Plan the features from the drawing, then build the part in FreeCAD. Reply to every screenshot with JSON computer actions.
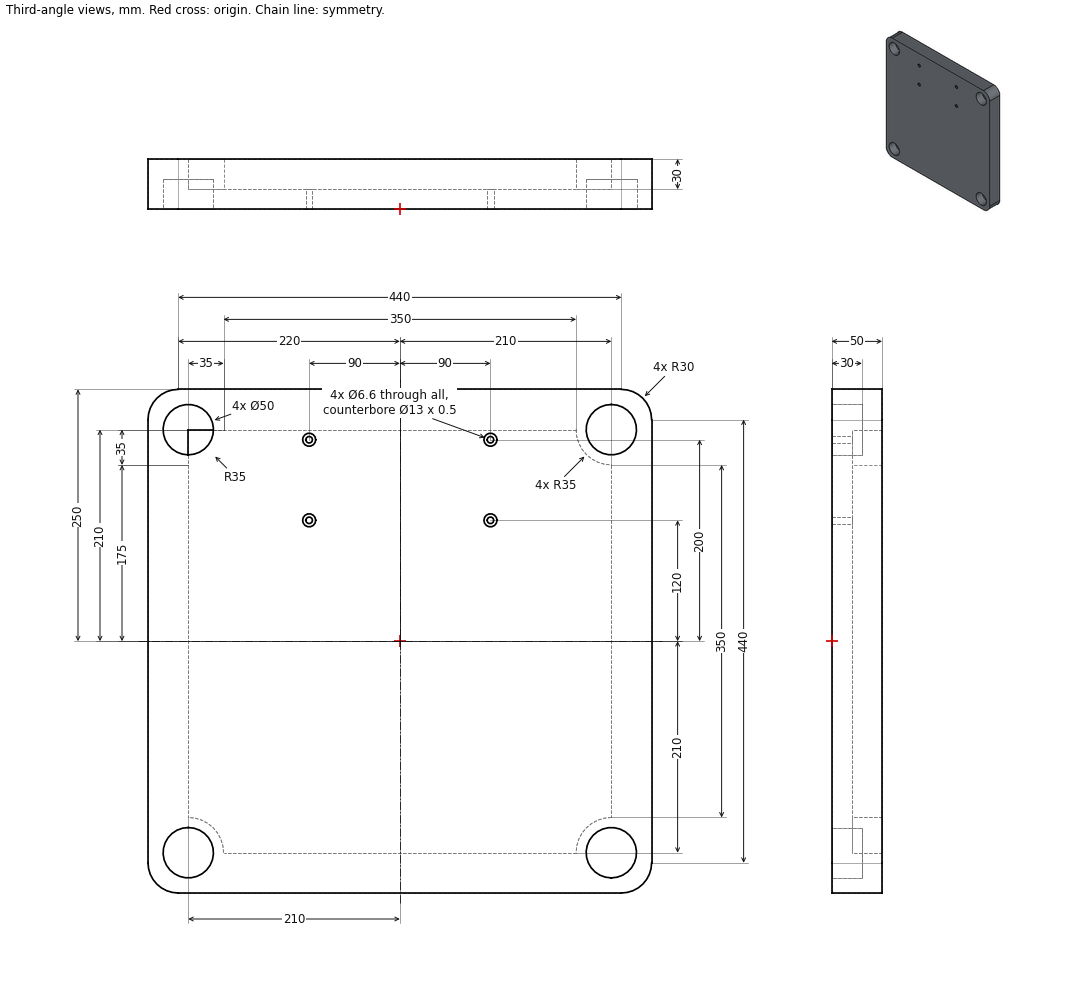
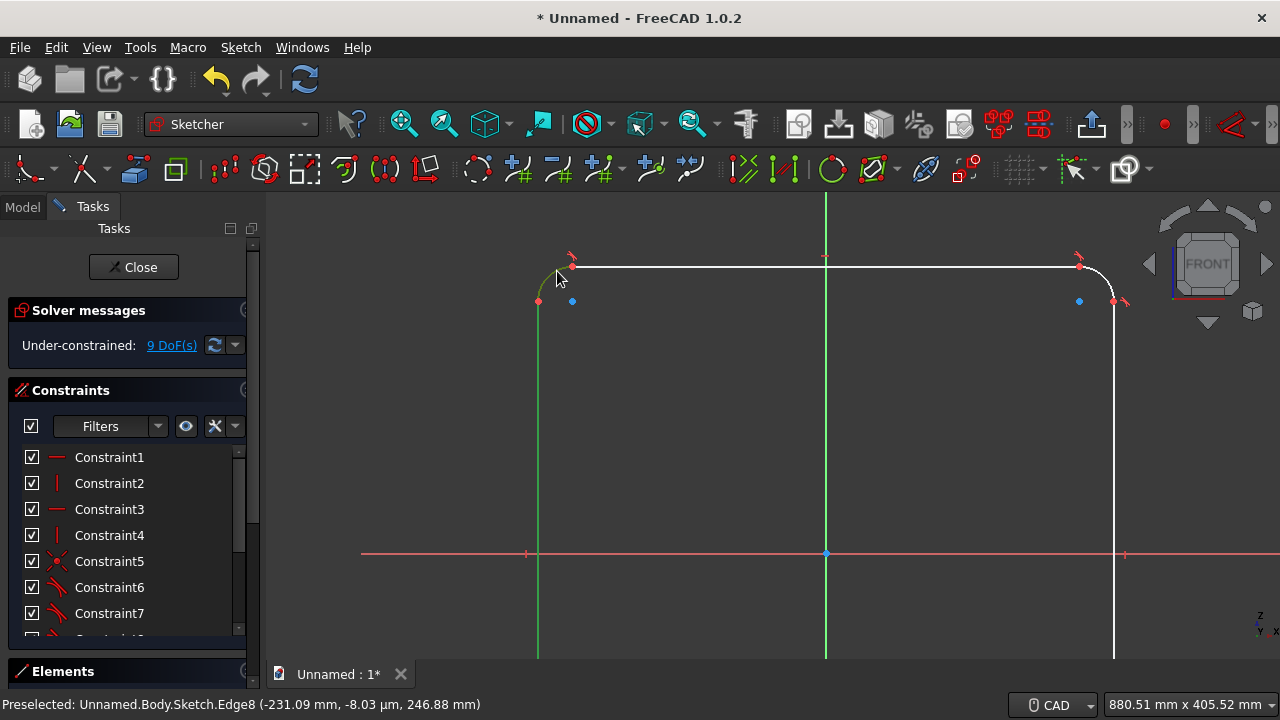
{"action": "key", "text": "t"}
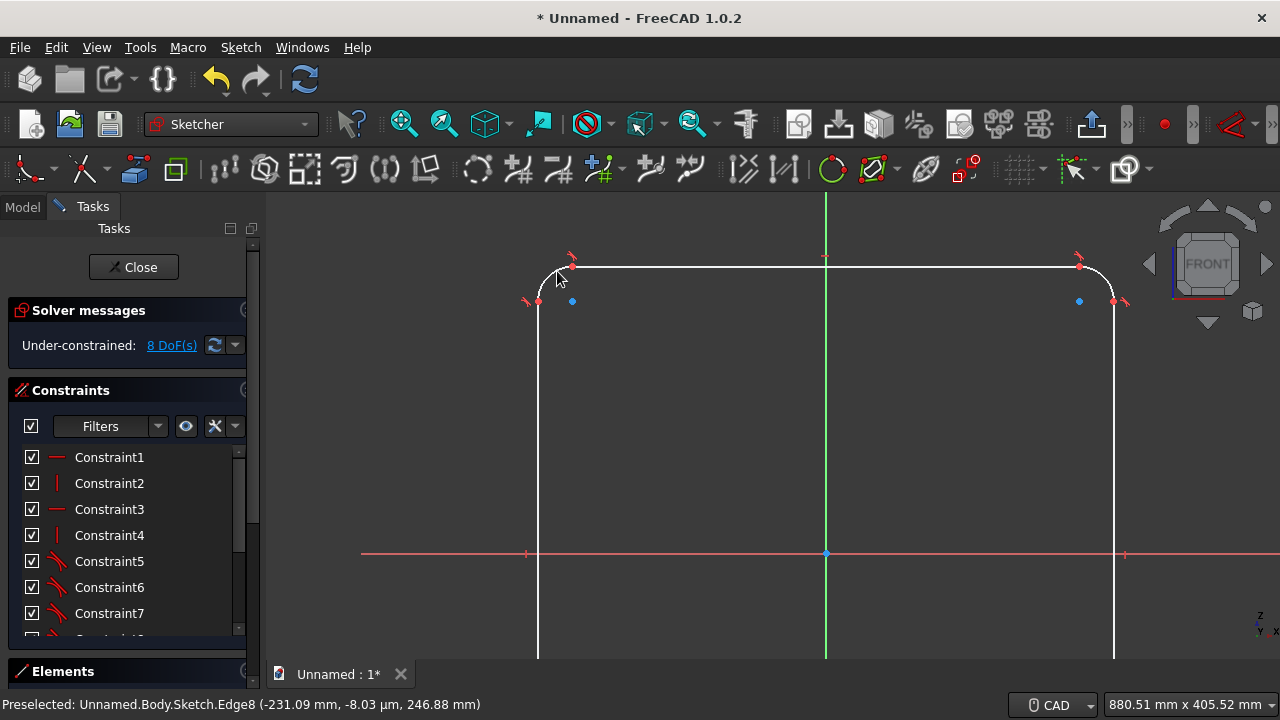
{"action": "left_click", "coordinate": [1110, 286]}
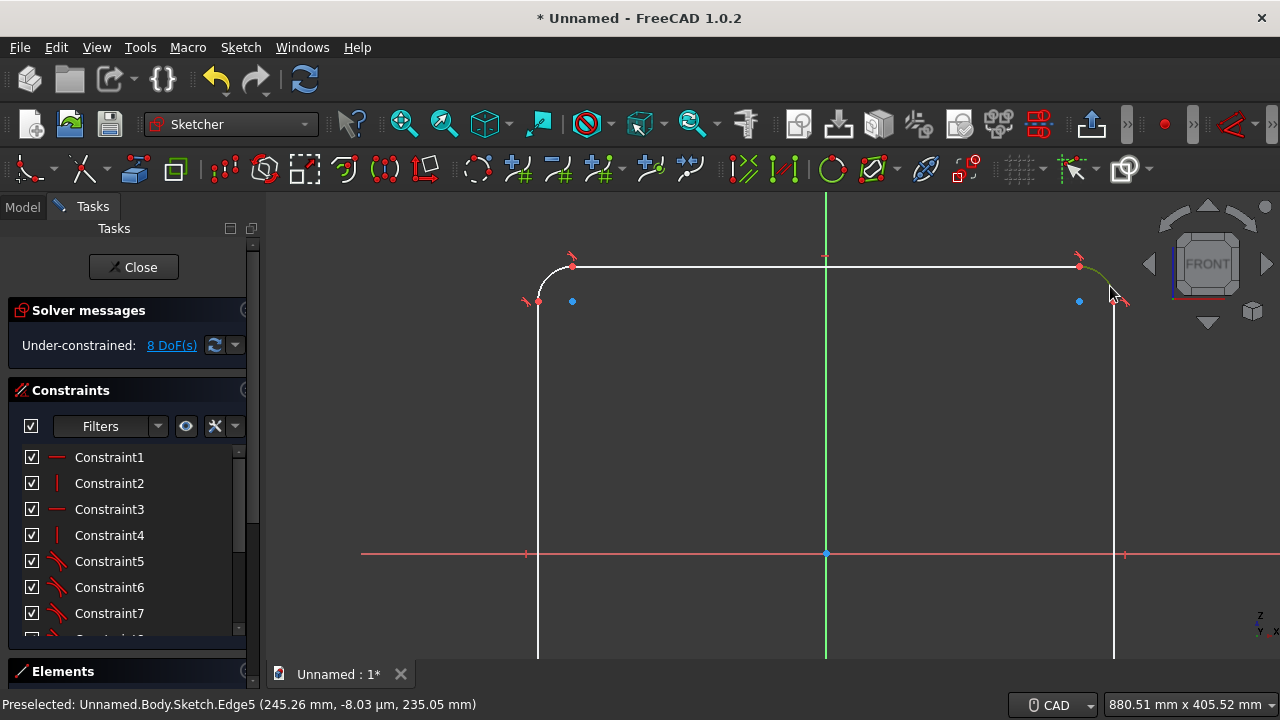
{"action": "scroll", "coordinate": [557, 270], "scroll_direction": "down", "scroll_amount": 3}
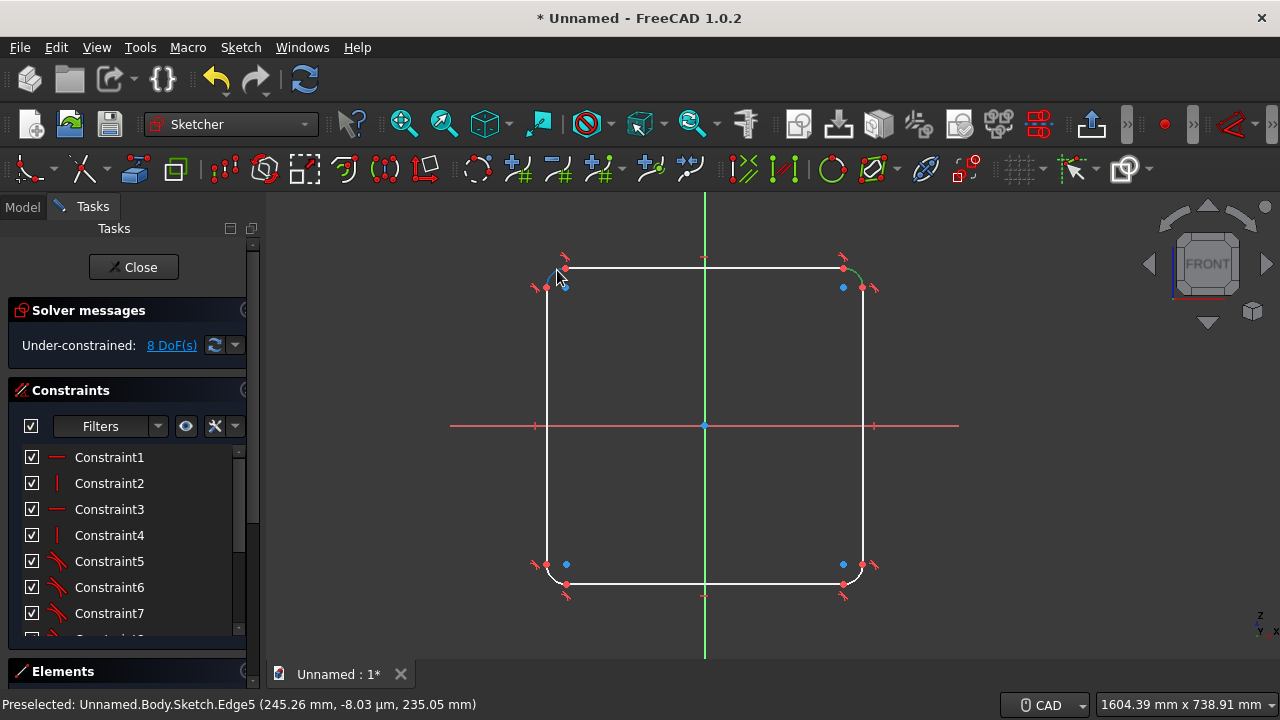
{"action": "scroll", "coordinate": [852, 582], "scroll_direction": "up", "scroll_amount": 3}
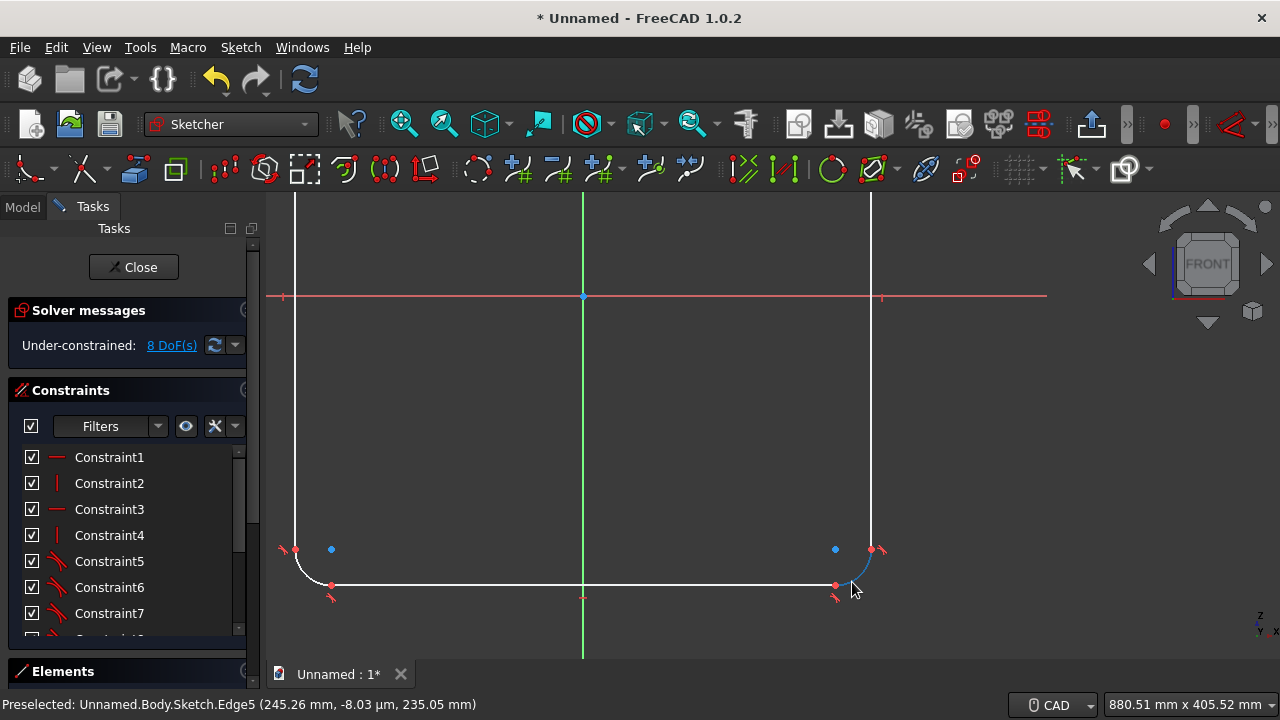
{"action": "left_click", "coordinate": [852, 582]}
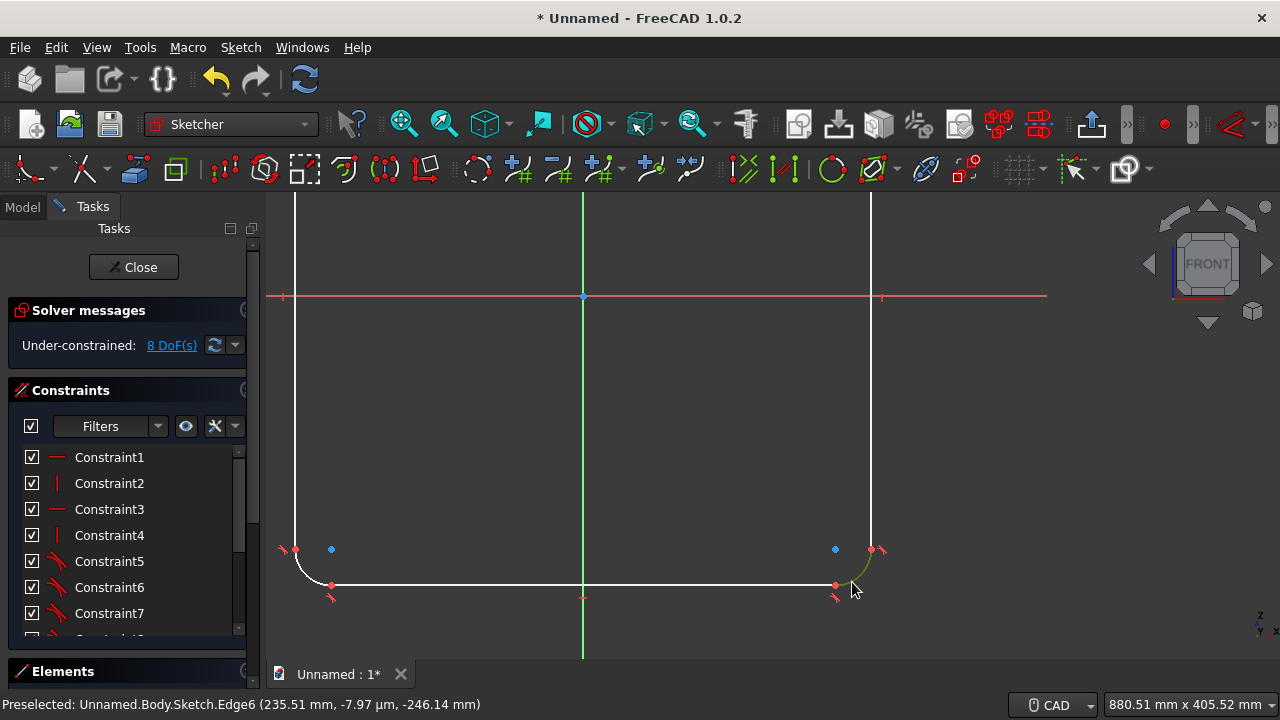
{"action": "left_click", "coordinate": [299, 566]}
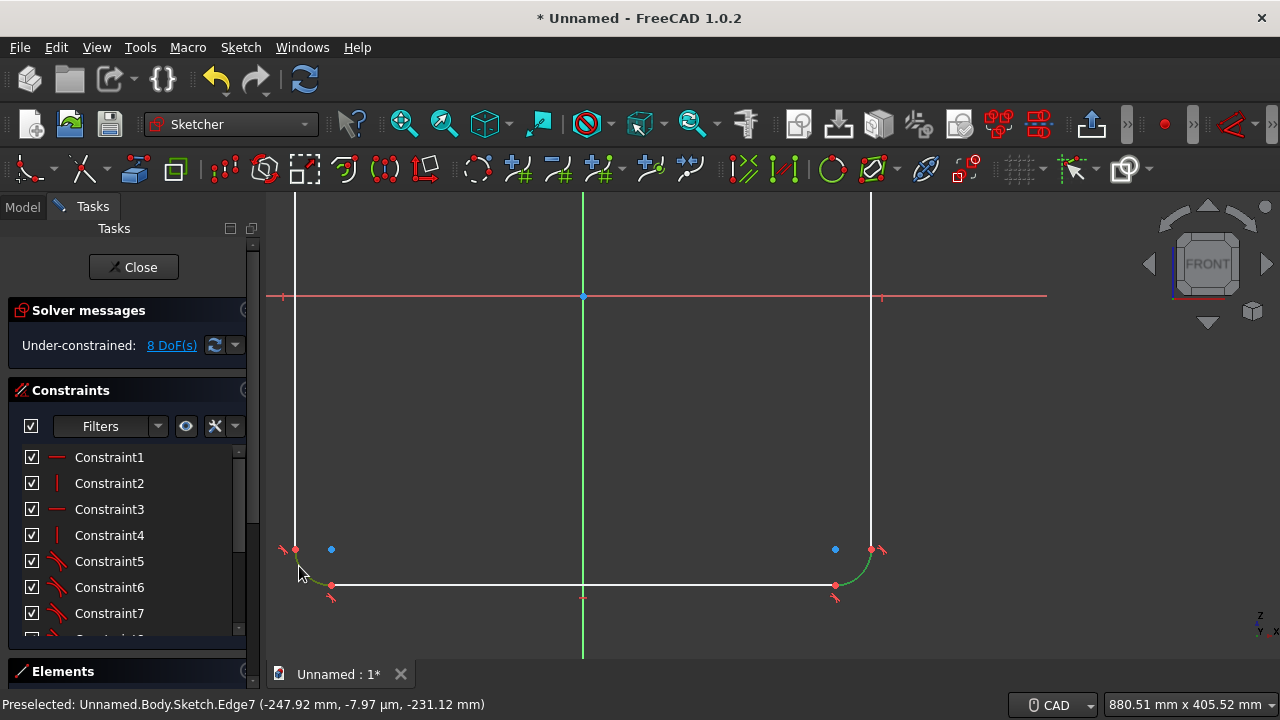
{"action": "scroll", "coordinate": [852, 582], "scroll_direction": "down", "scroll_amount": 3}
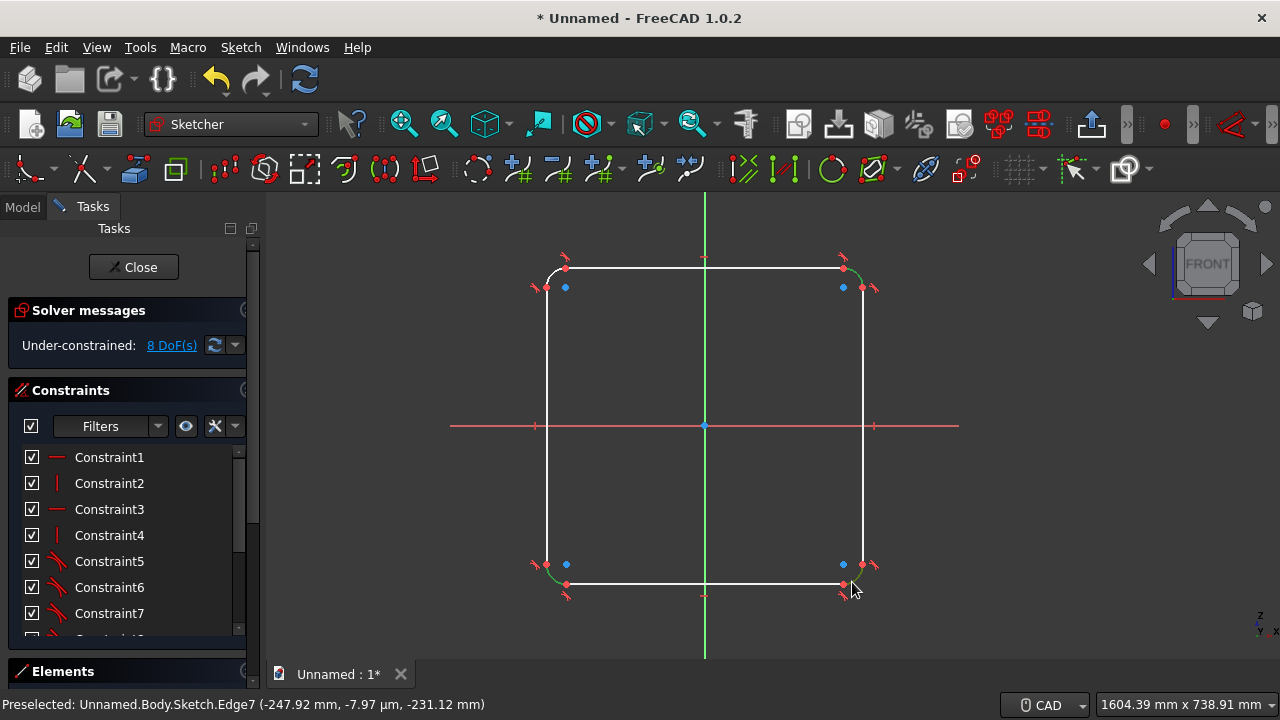
{"action": "scroll", "coordinate": [557, 270], "scroll_direction": "up", "scroll_amount": 3}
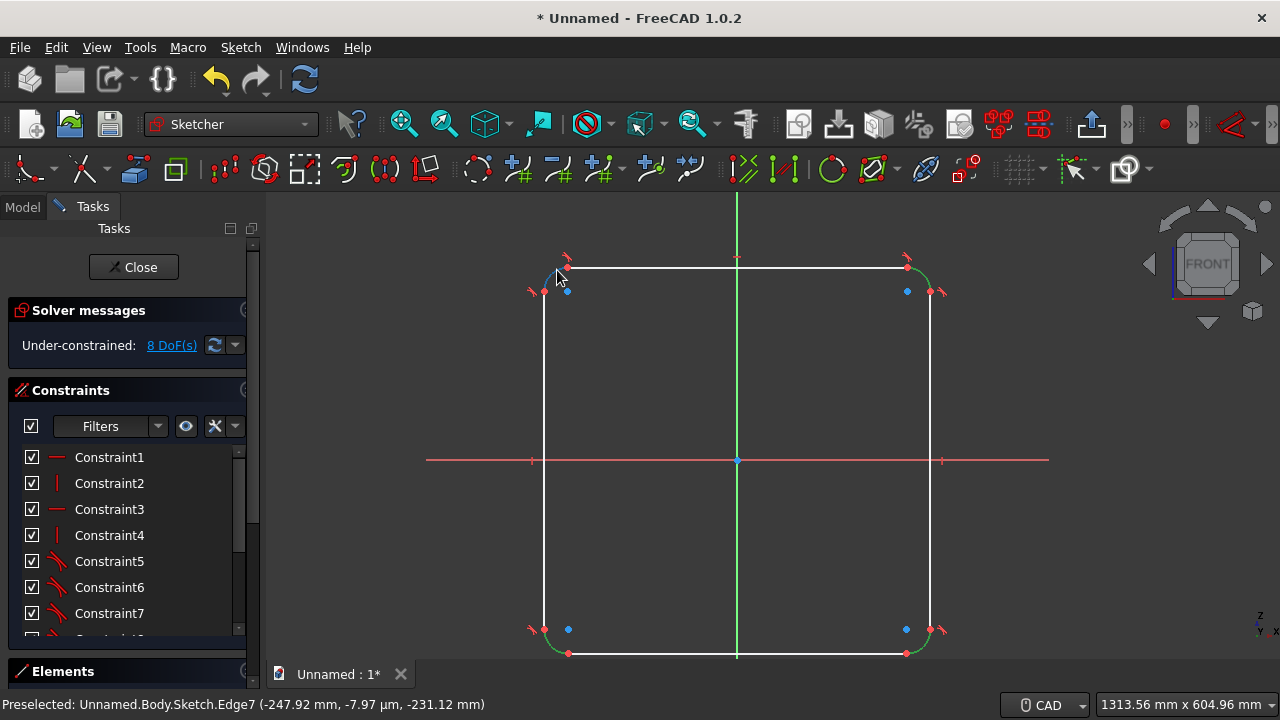
{"action": "left_click", "coordinate": [557, 270]}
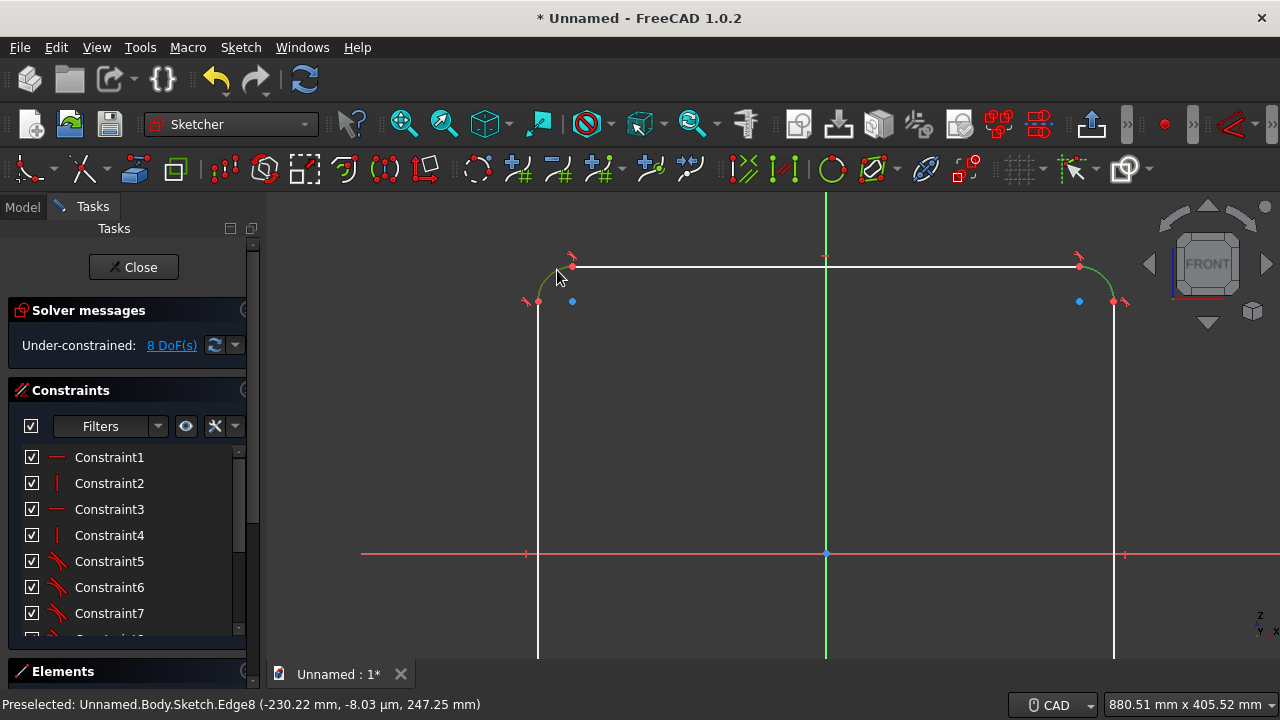
{"action": "key", "text": "e"}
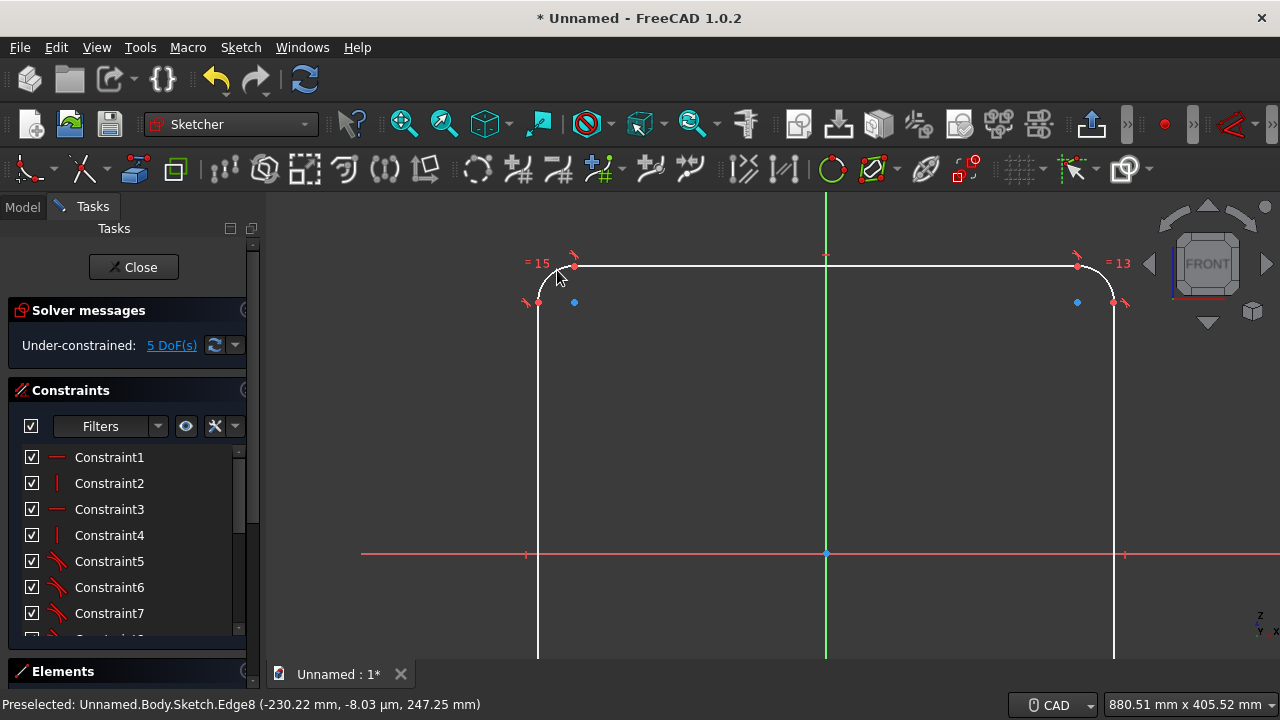
{"action": "left_click", "coordinate": [1232, 124]}